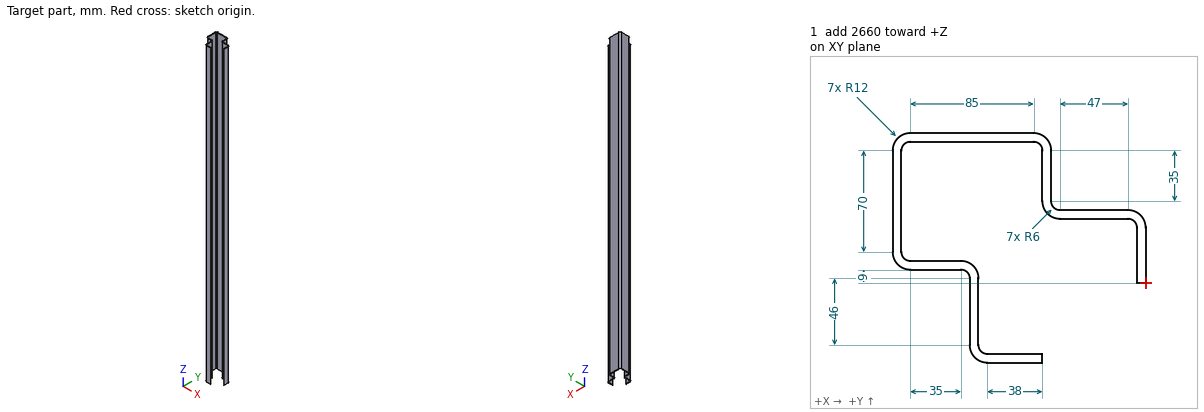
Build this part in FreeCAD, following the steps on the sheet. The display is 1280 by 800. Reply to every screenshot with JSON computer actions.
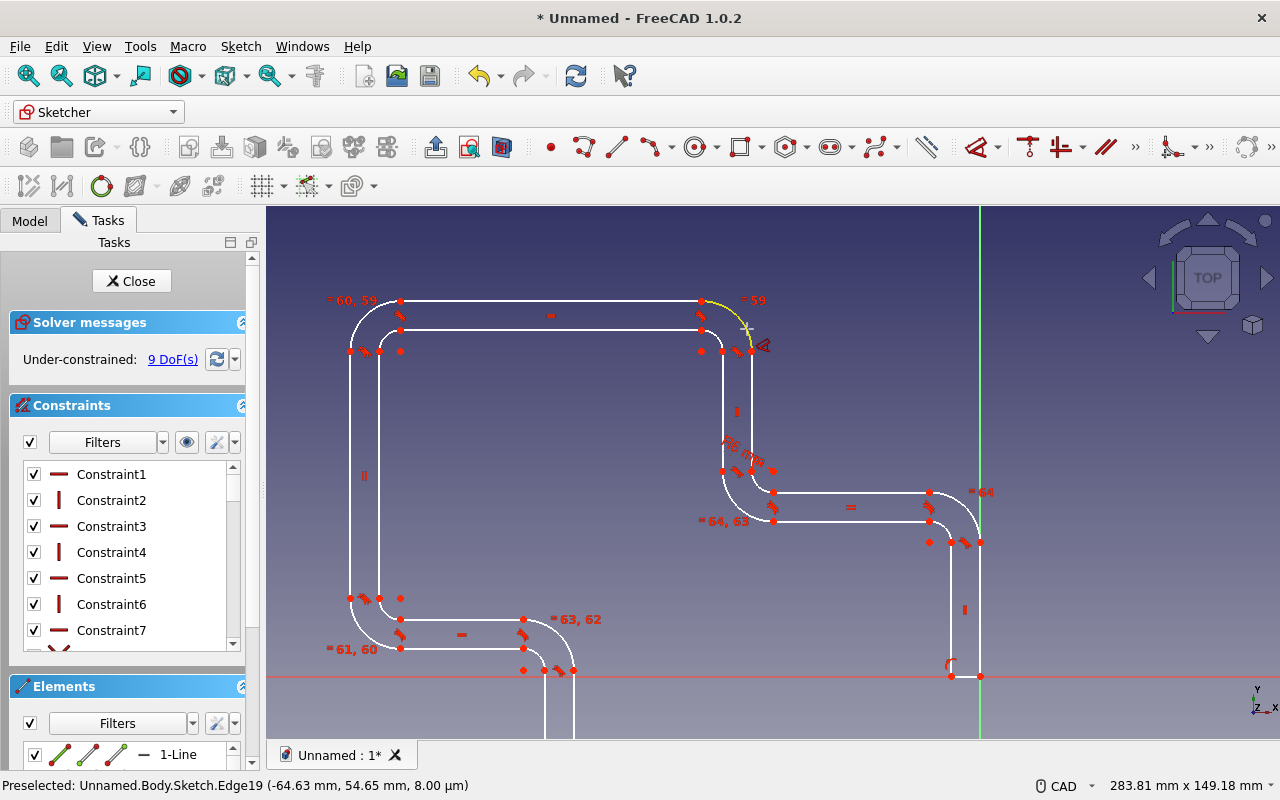
{"action": "left_click", "coordinate": [746, 329]}
{"action": "left_click", "coordinate": [775, 315]}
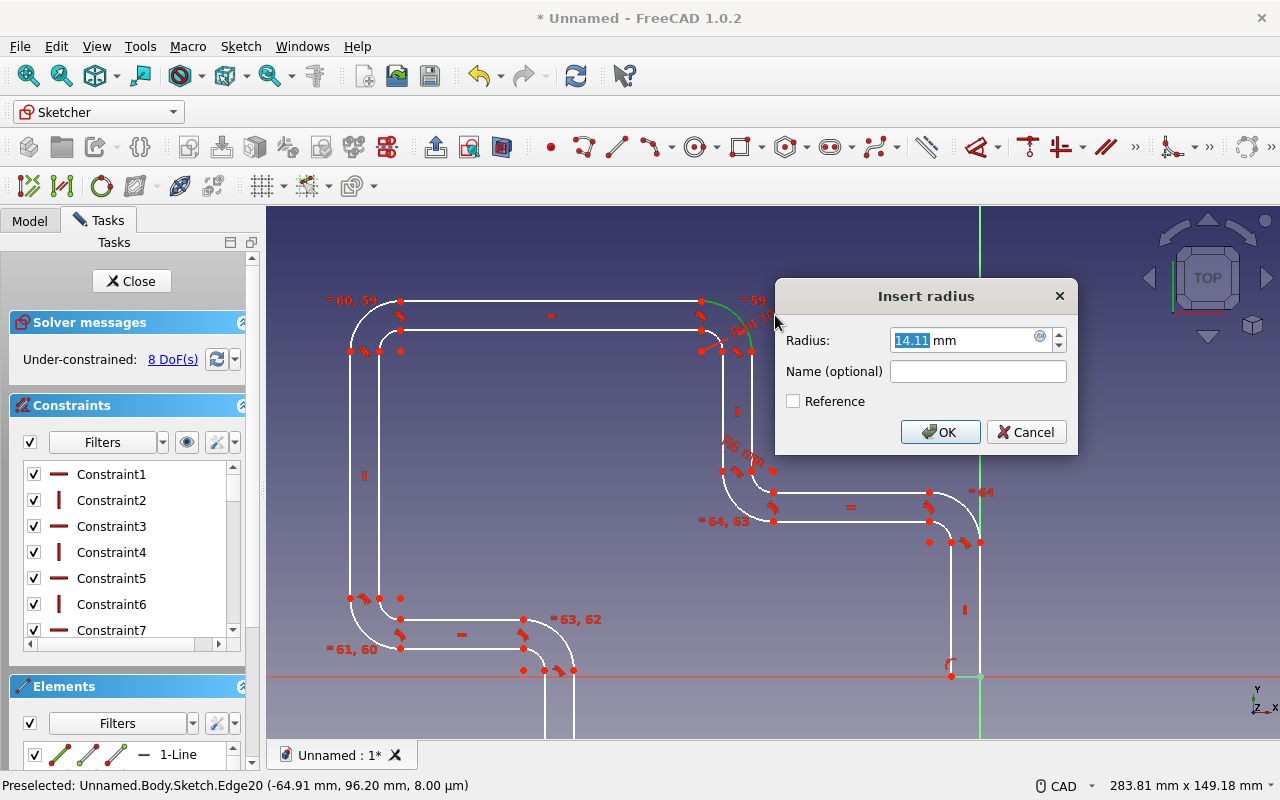
{"action": "type", "text": "12"}
{"action": "key", "text": "Return"}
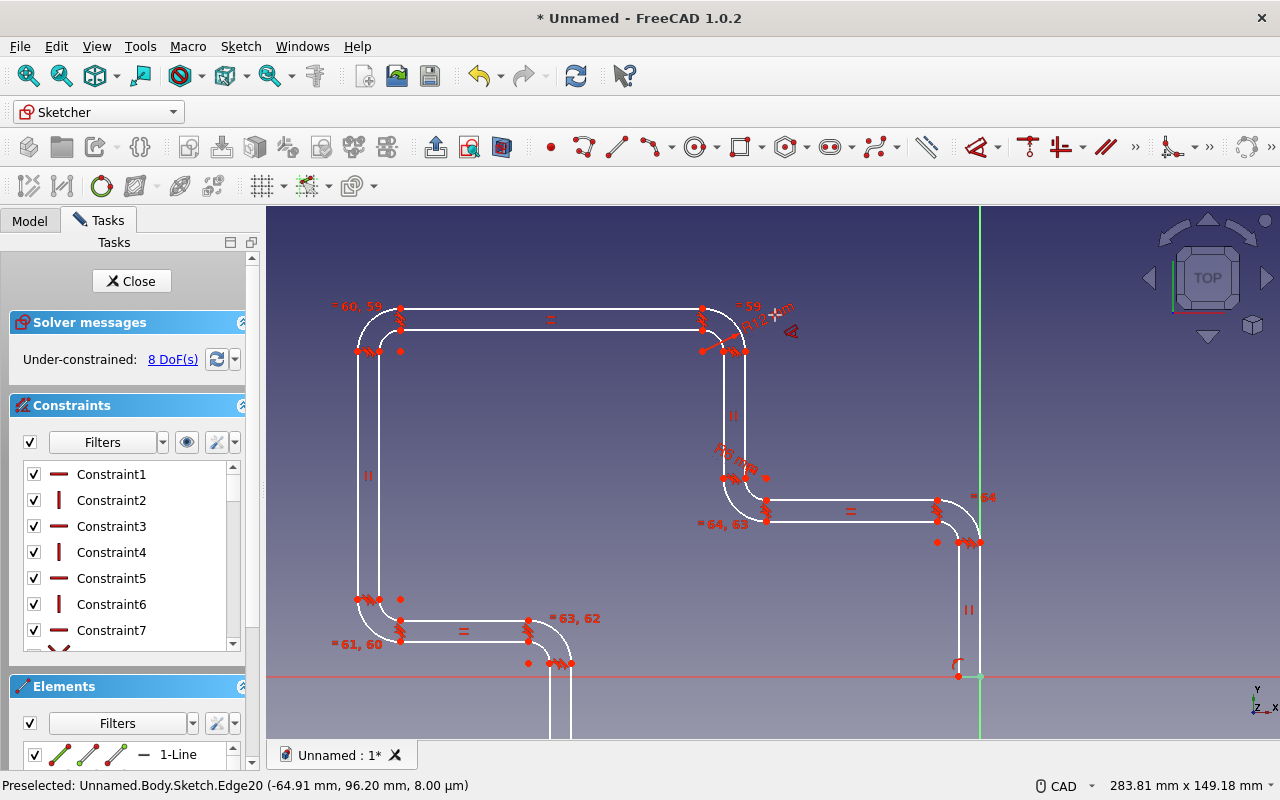
{"action": "left_click", "coordinate": [886, 500]}
{"action": "left_click", "coordinate": [852, 466]}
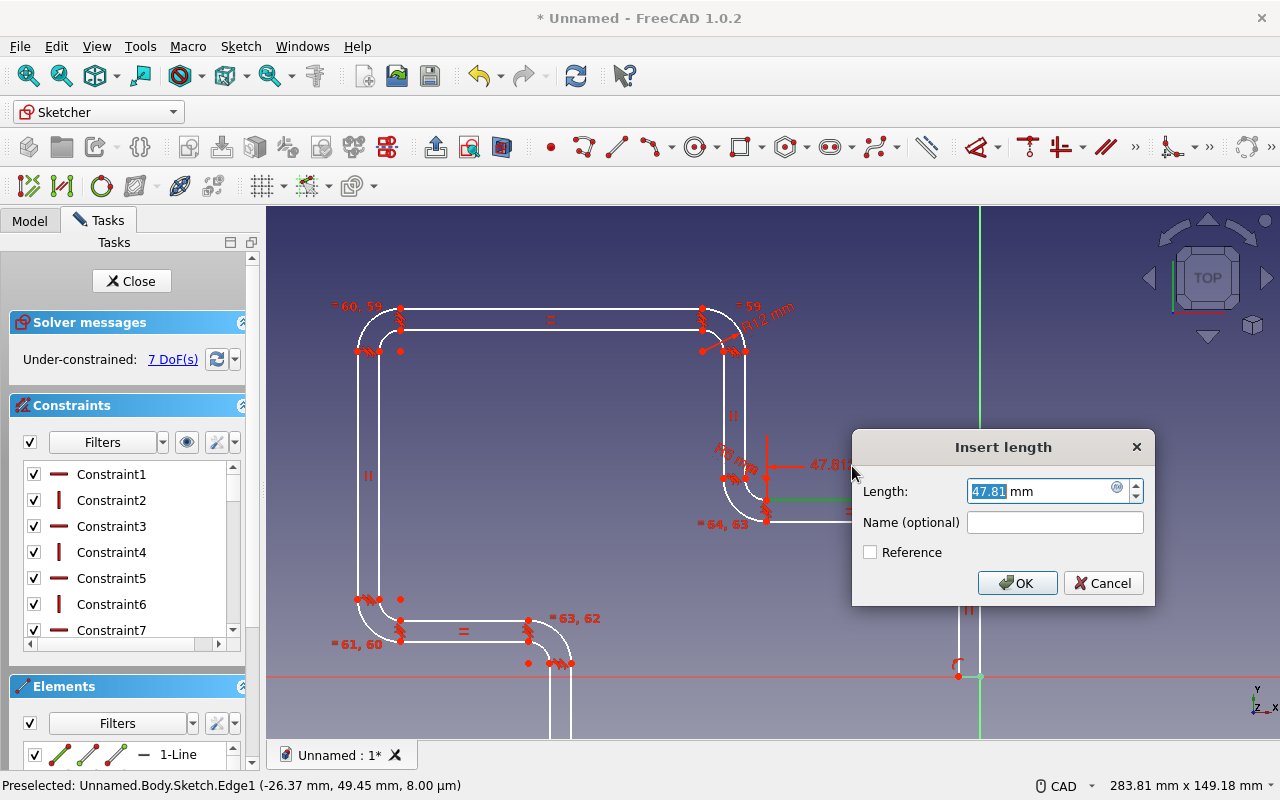
{"action": "type", "text": "47"}
{"action": "key", "text": "Return"}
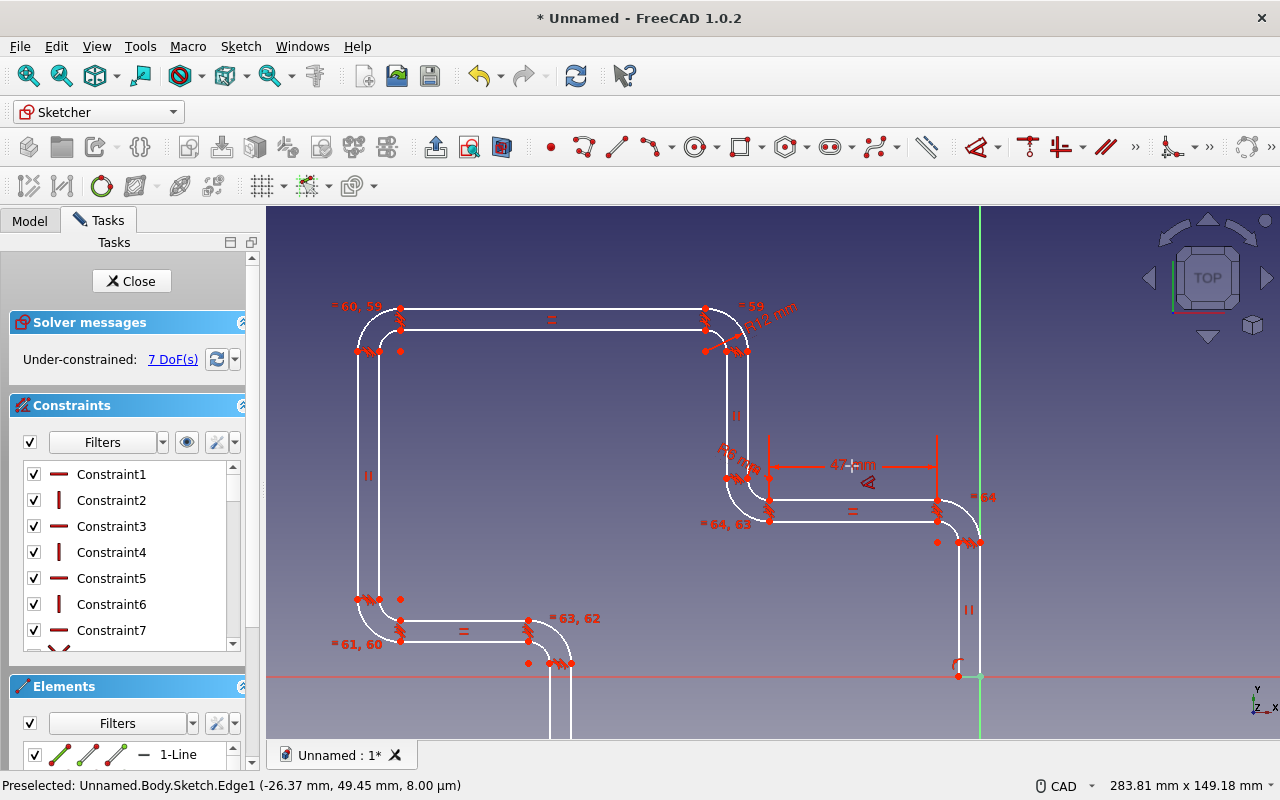
{"action": "left_click", "coordinate": [748, 441]}
{"action": "left_click", "coordinate": [782, 415]}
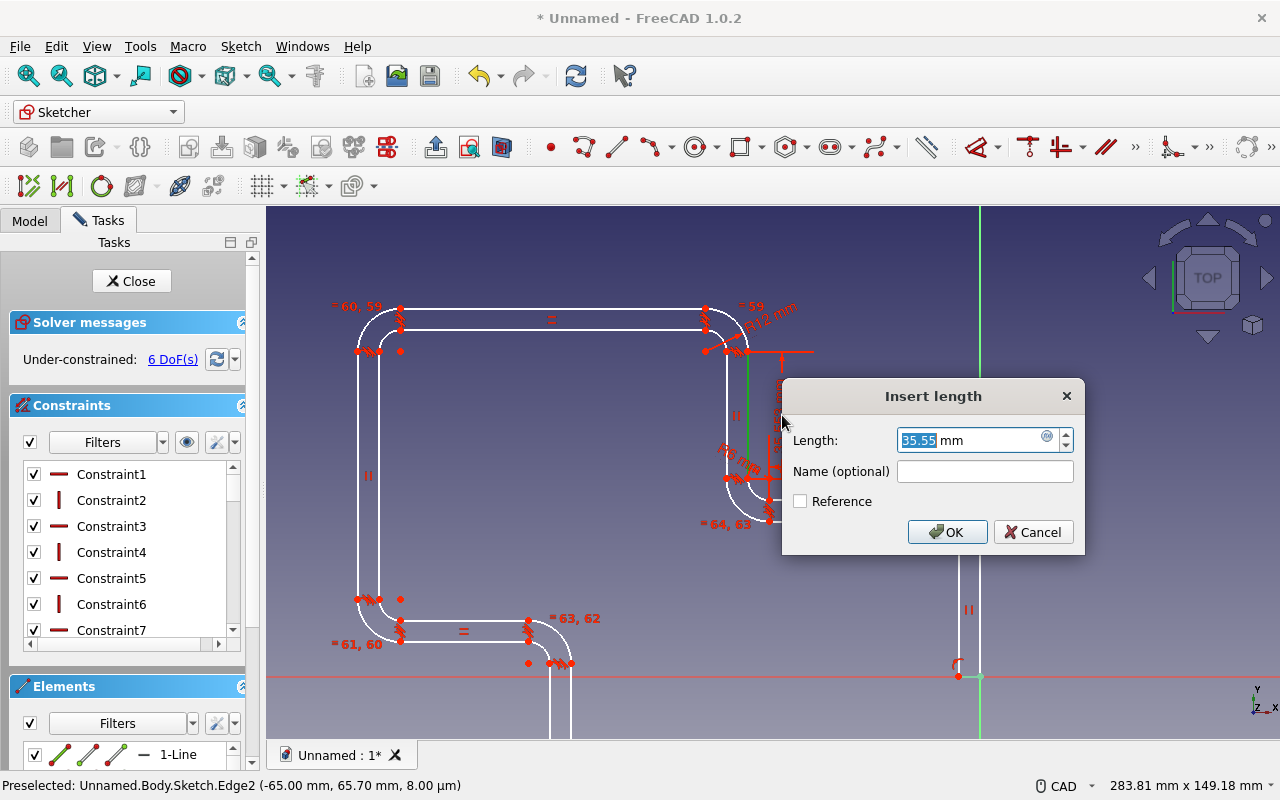
{"action": "type", "text": "35"}
{"action": "key", "text": "Return"}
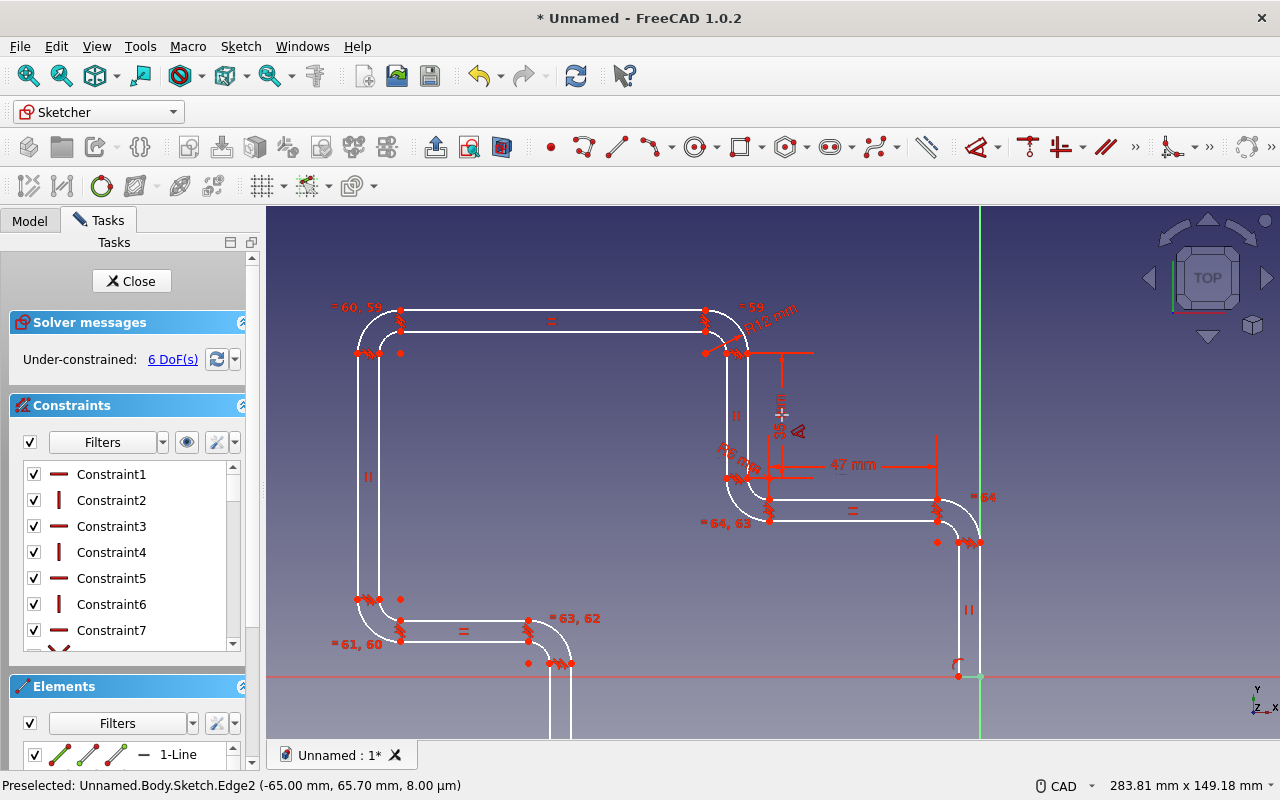
{"action": "left_click", "coordinate": [614, 310]}
{"action": "left_click", "coordinate": [553, 276]}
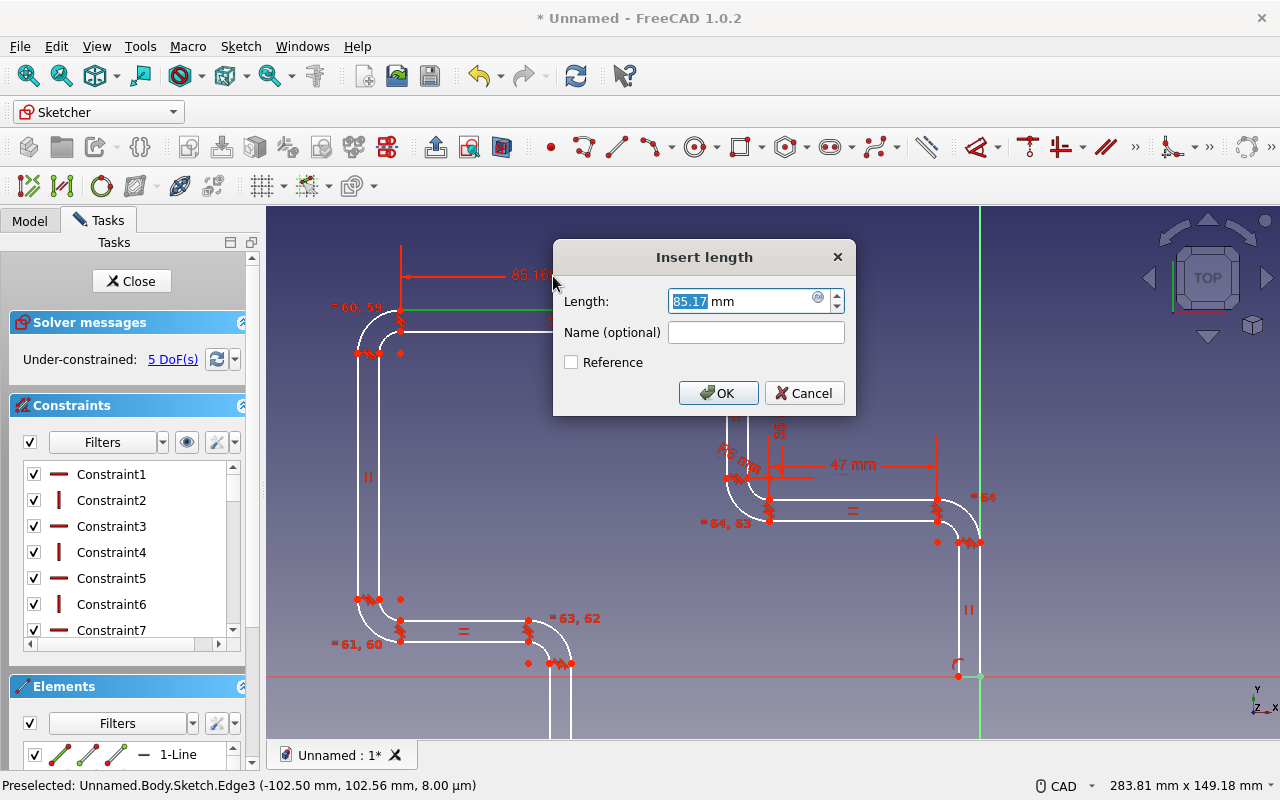
{"action": "type", "text": "85"}
{"action": "key", "text": "Return"}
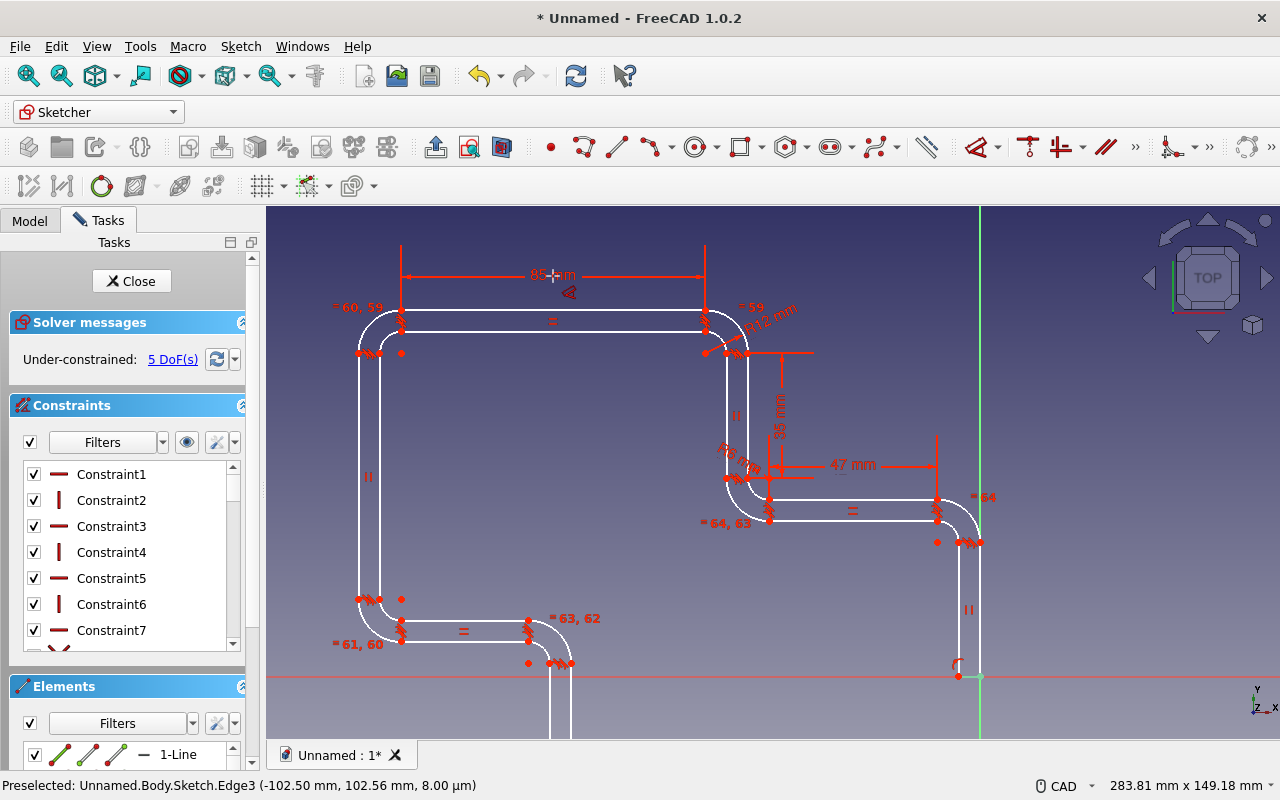
{"action": "left_click", "coordinate": [359, 427]}
{"action": "left_click", "coordinate": [325, 476]}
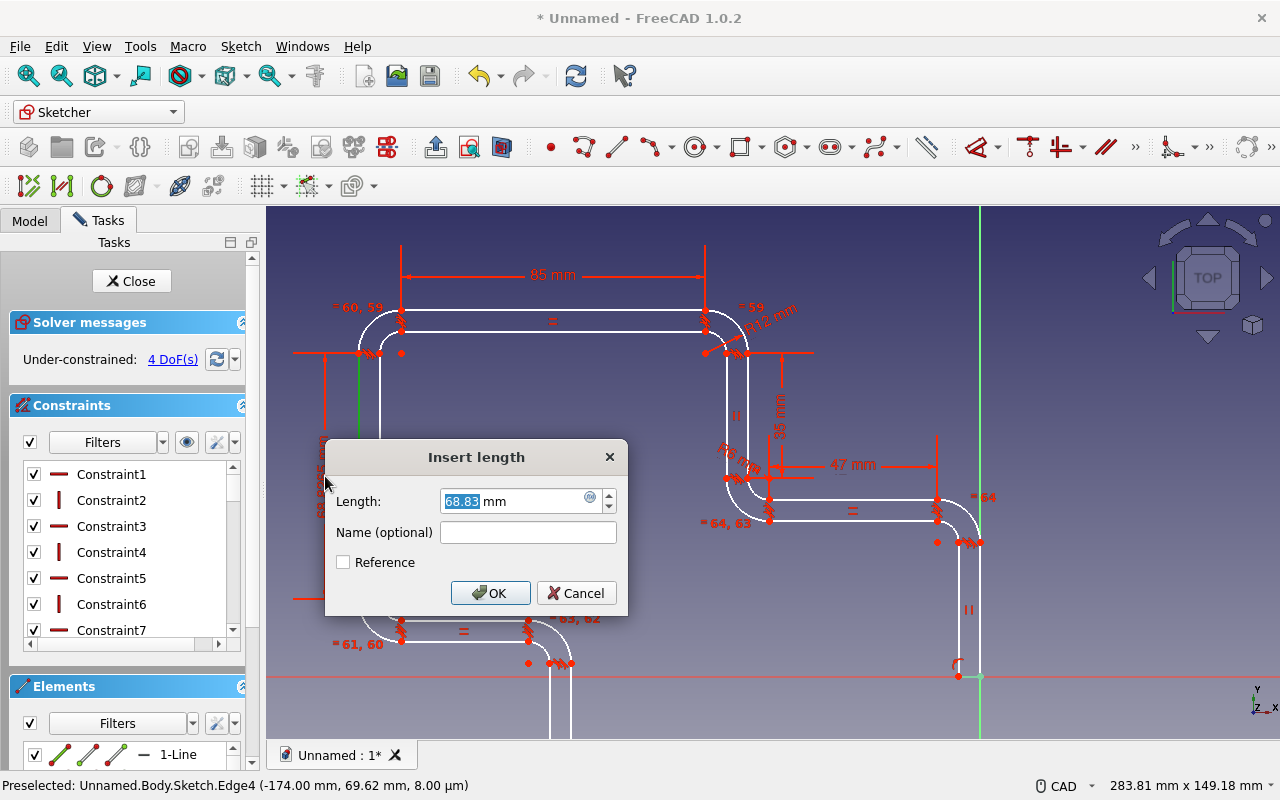
{"action": "type", "text": "70"}
{"action": "key", "text": "Return"}